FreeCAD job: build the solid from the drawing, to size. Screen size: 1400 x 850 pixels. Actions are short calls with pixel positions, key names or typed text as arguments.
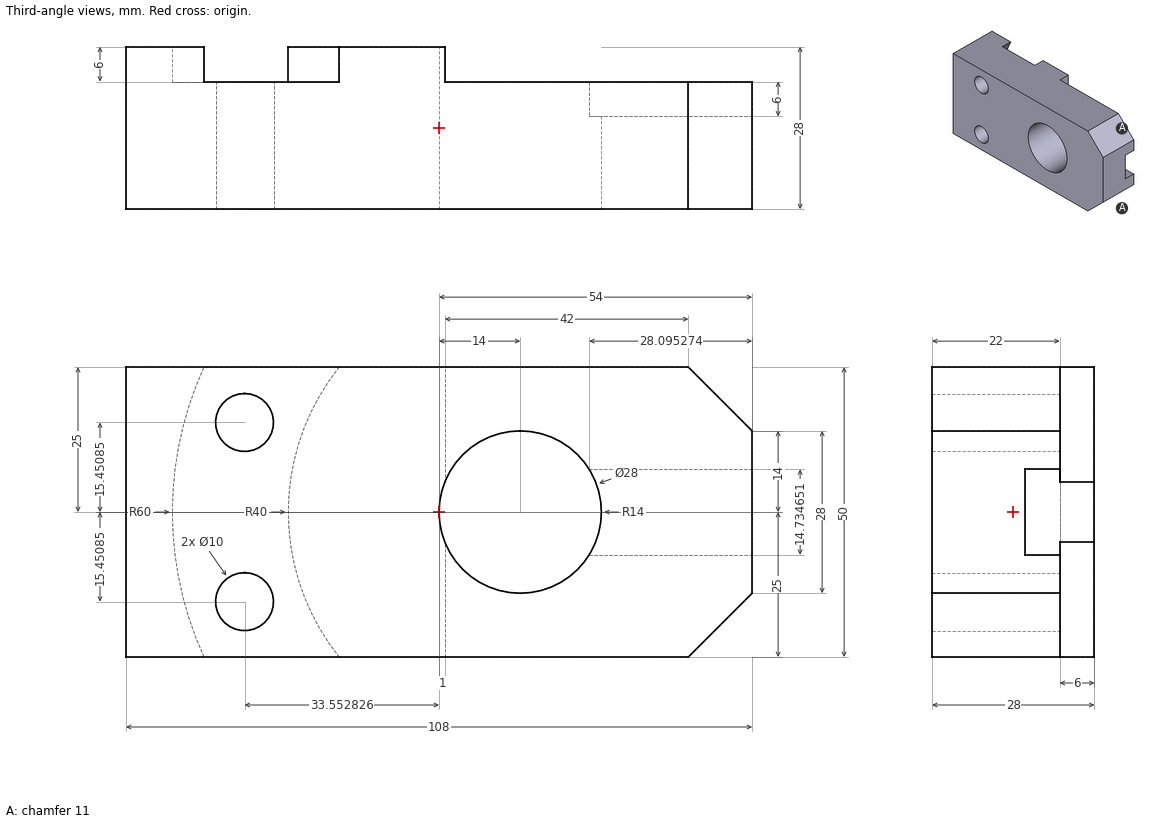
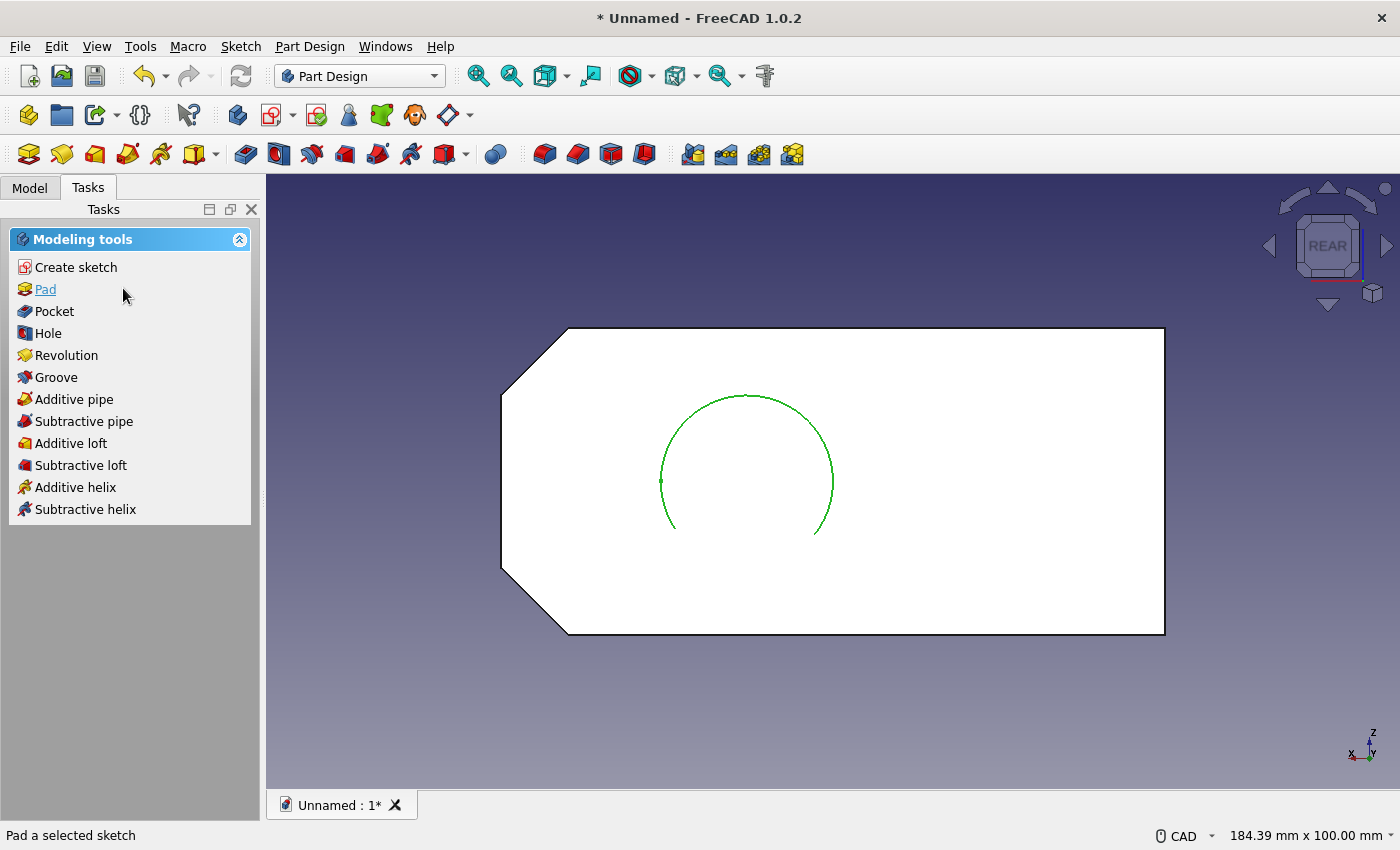
click(246, 154)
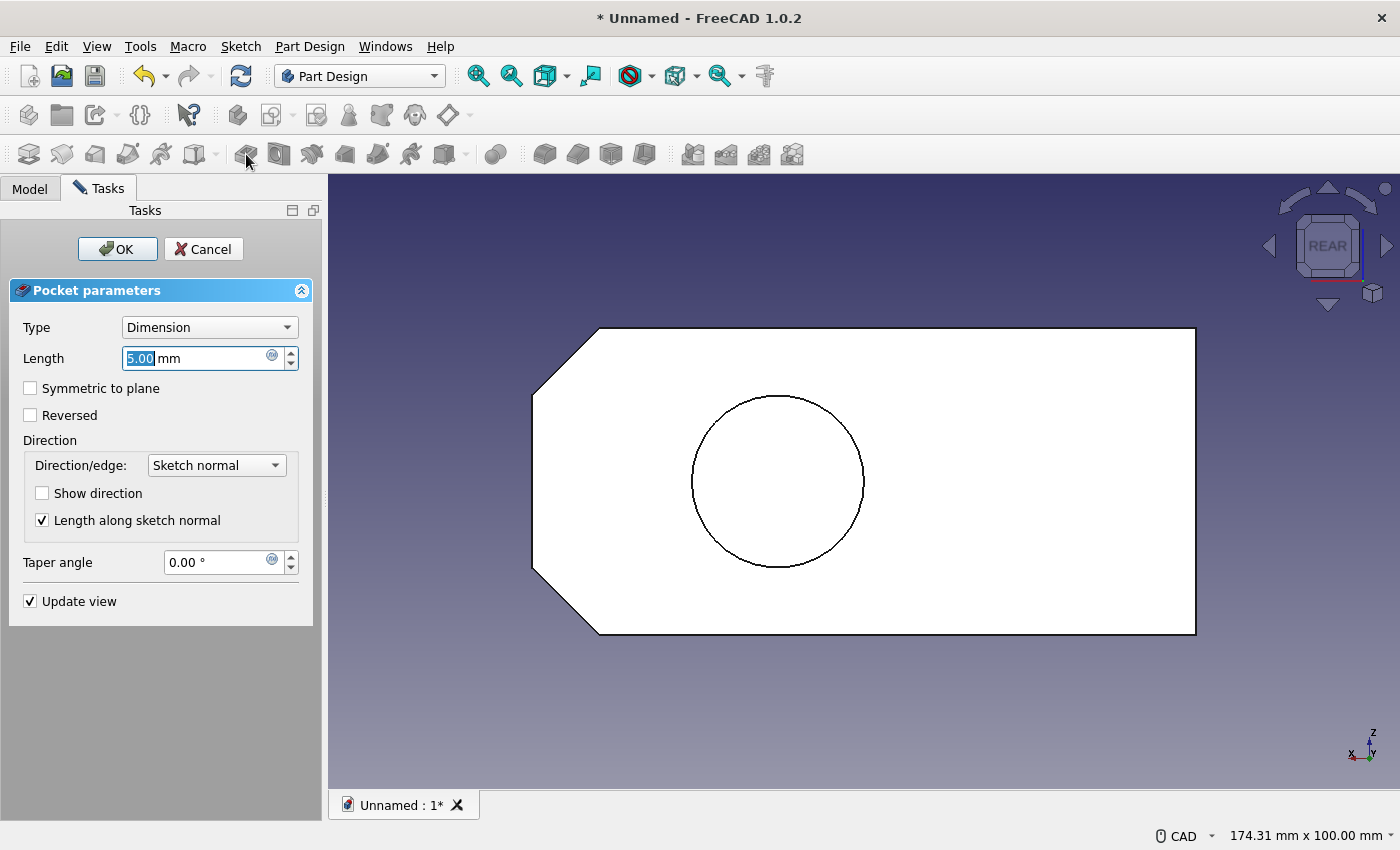
text(28)
key(Tab)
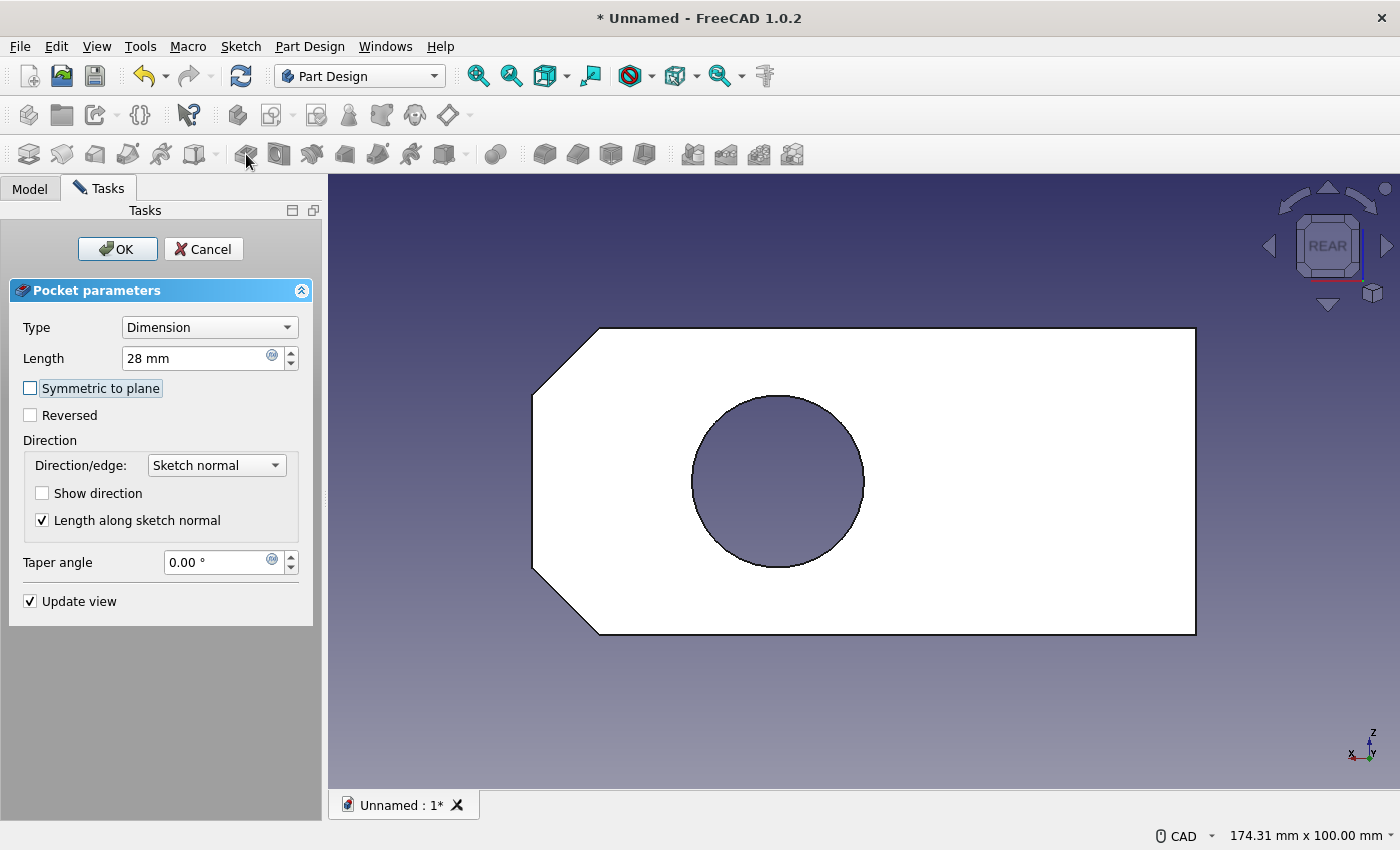
click(118, 249)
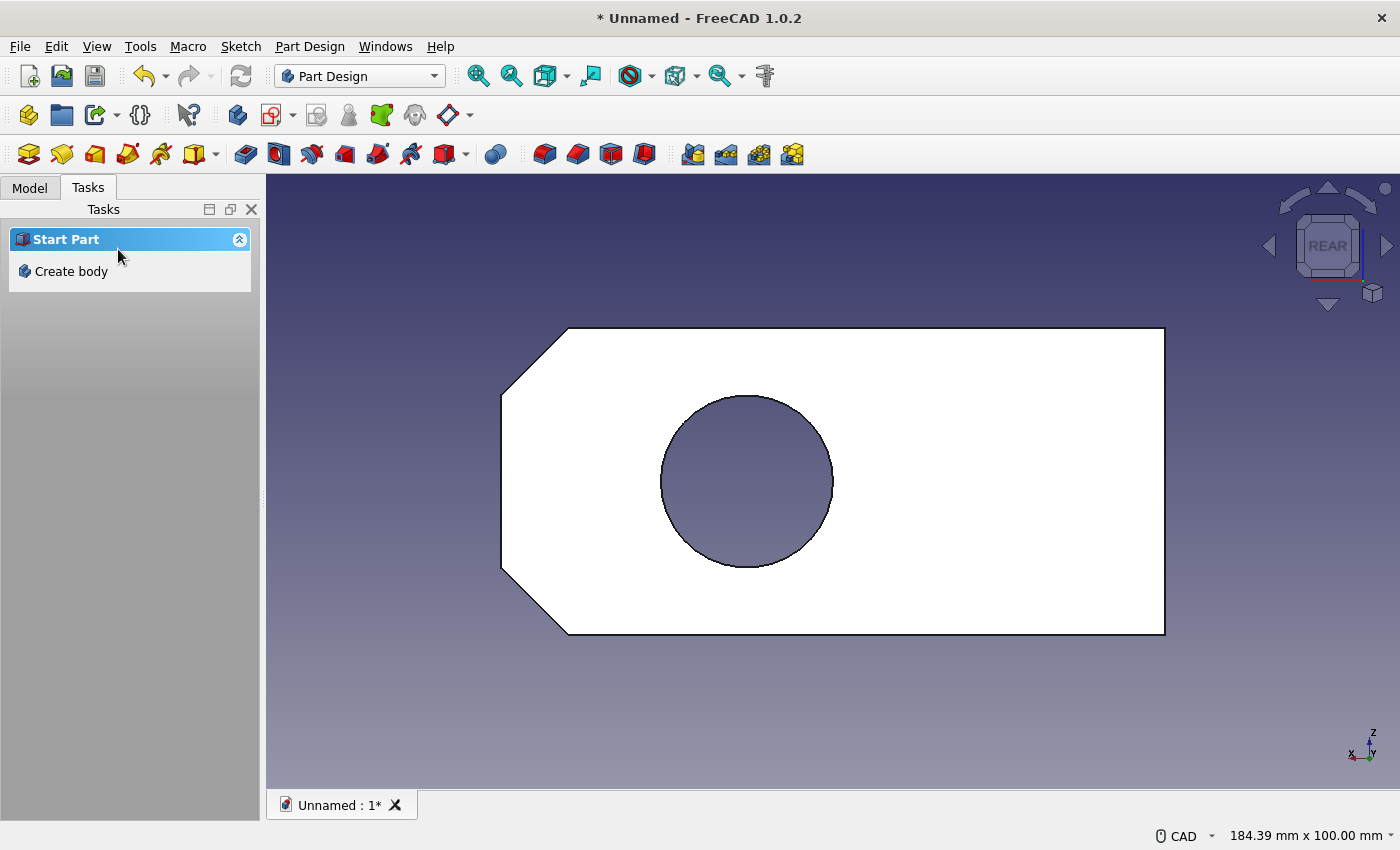
click(1023, 480)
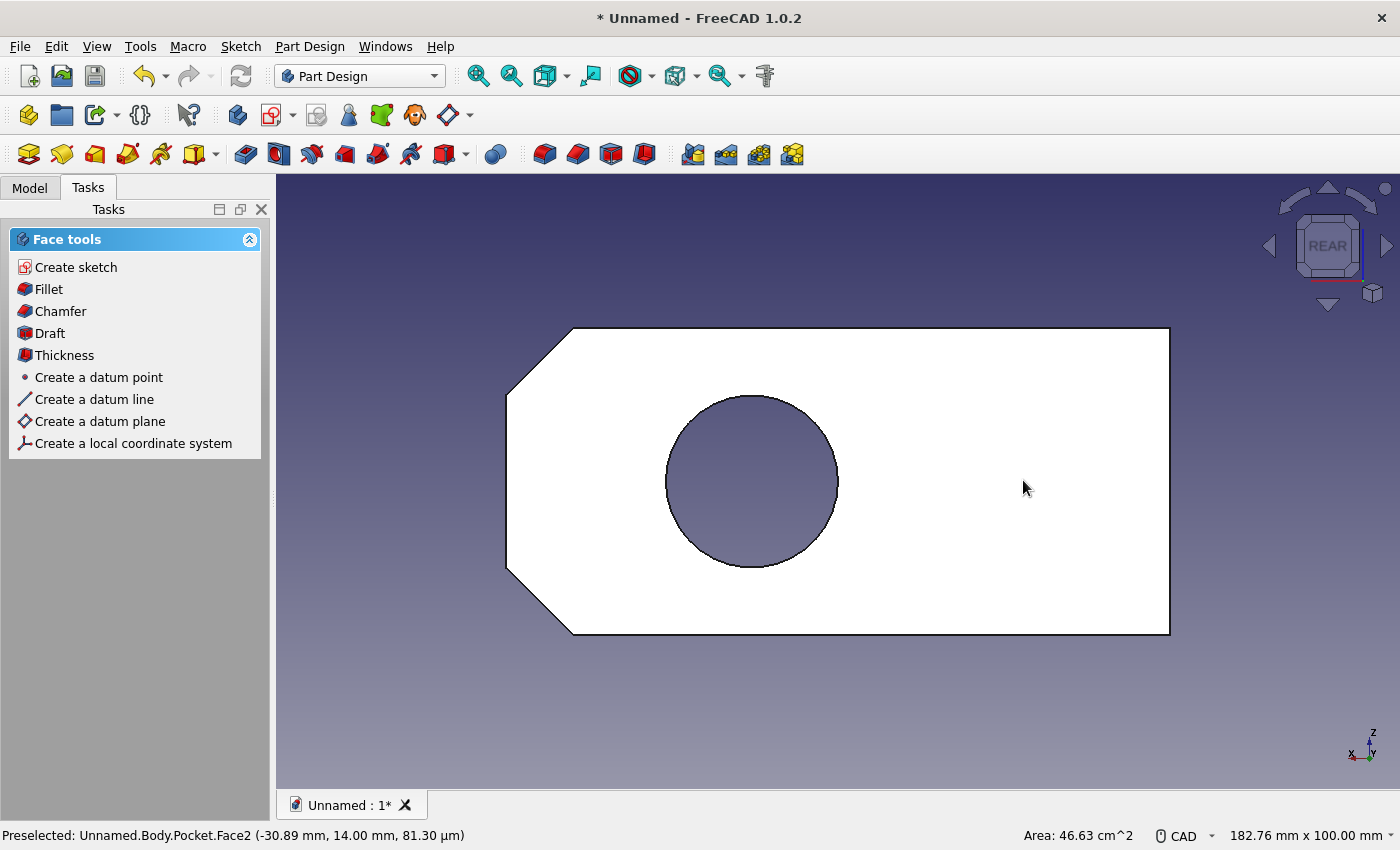
click(270, 116)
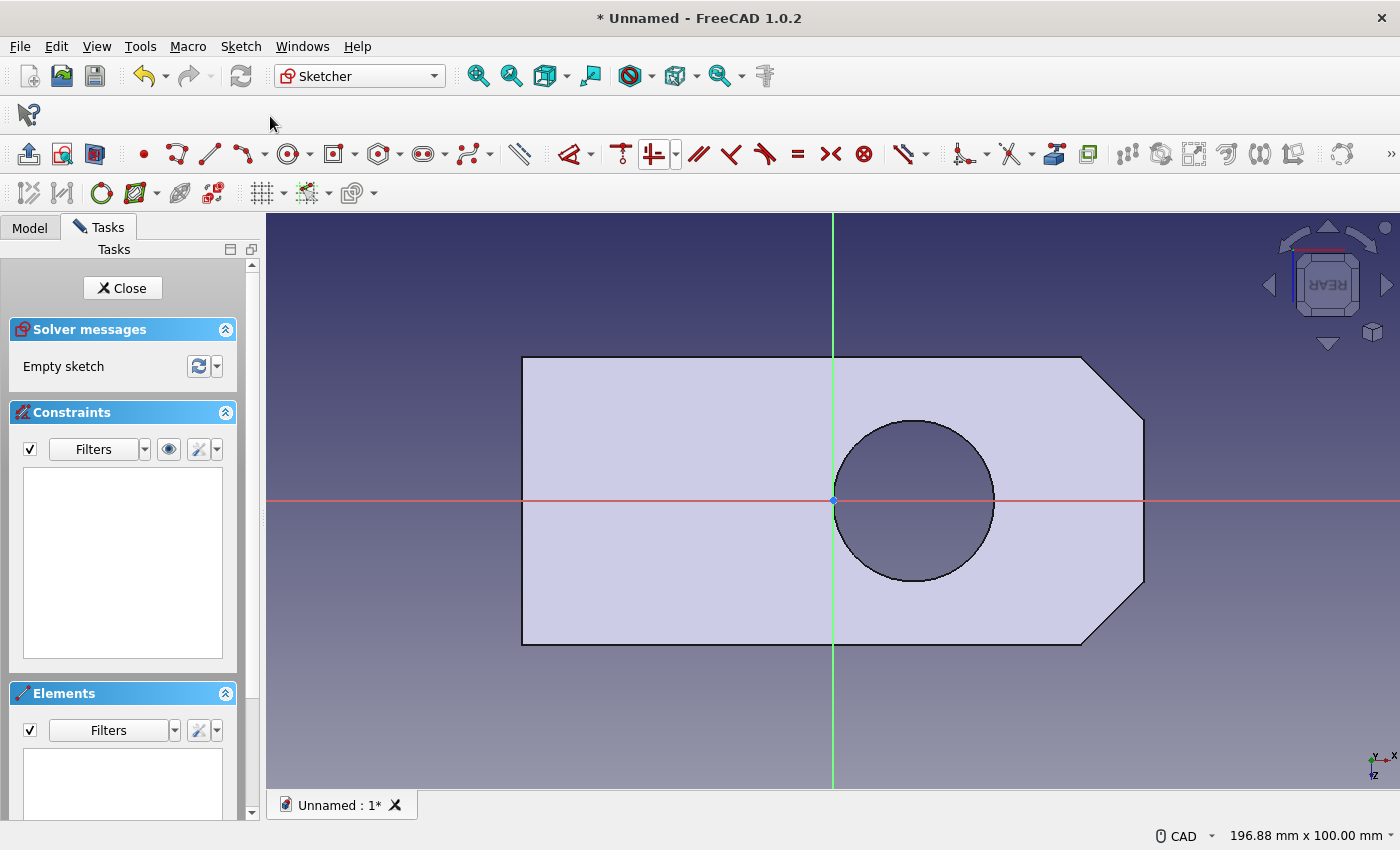
click(177, 154)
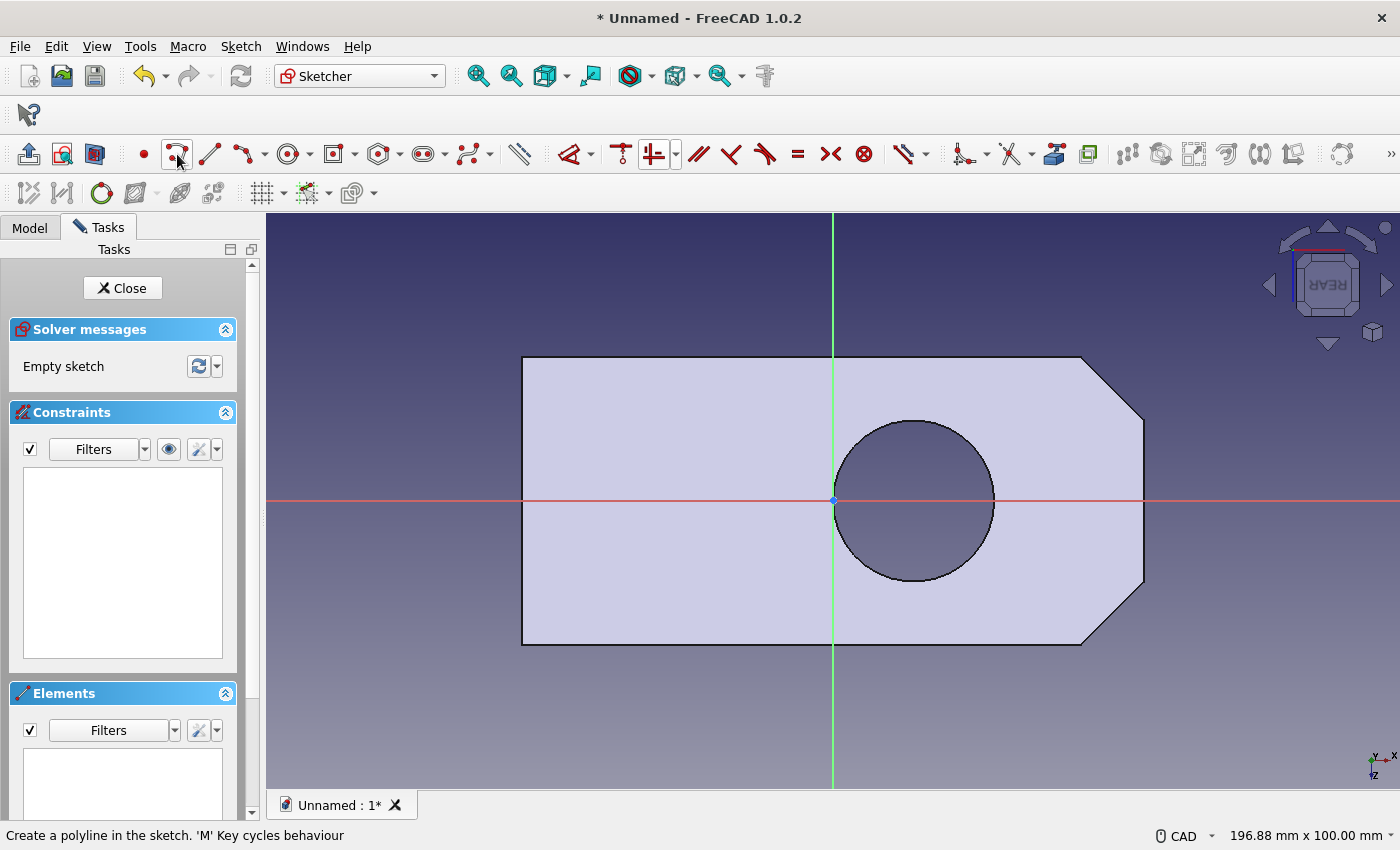
scroll(839, 357, up, 6)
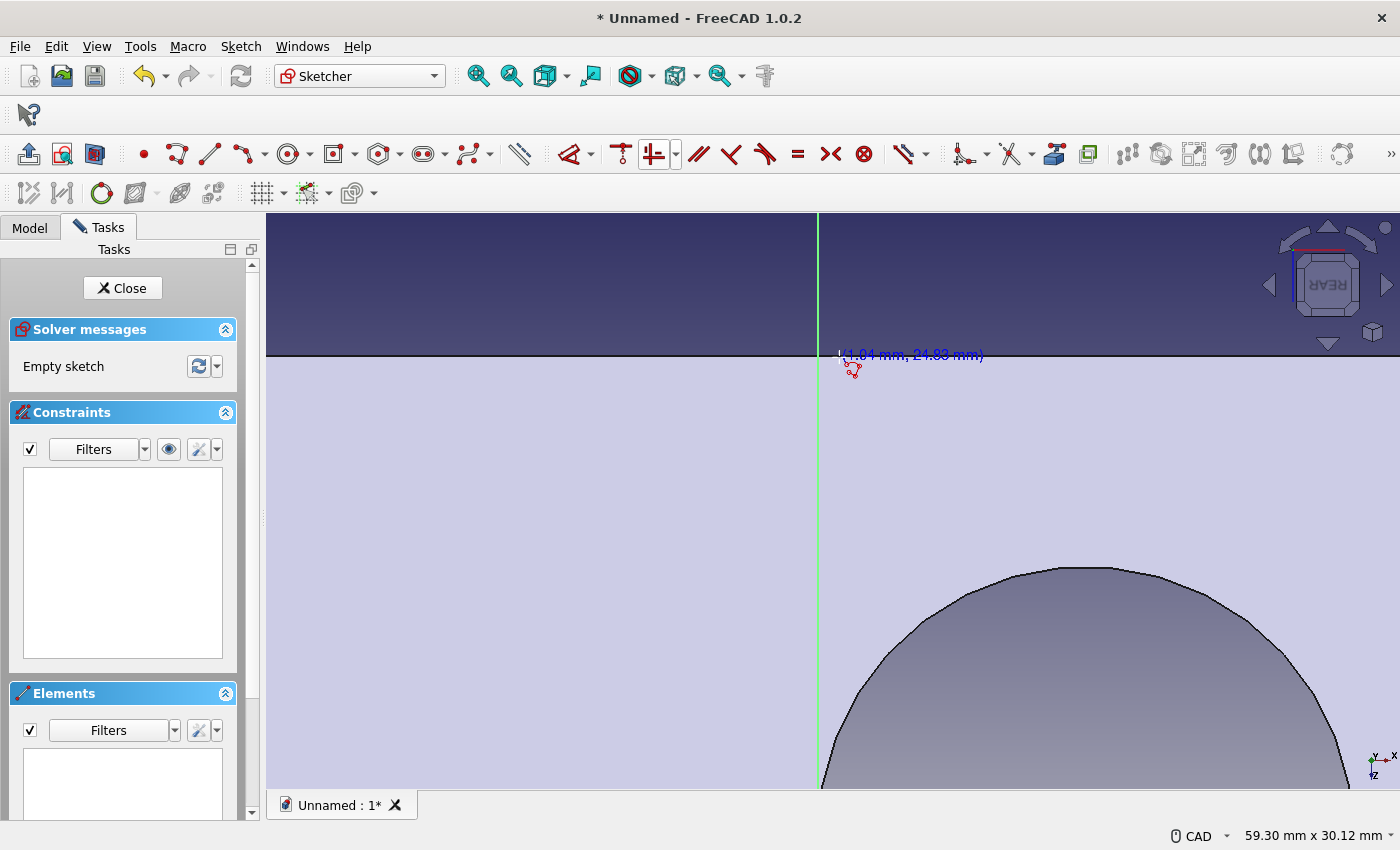
click(837, 356)